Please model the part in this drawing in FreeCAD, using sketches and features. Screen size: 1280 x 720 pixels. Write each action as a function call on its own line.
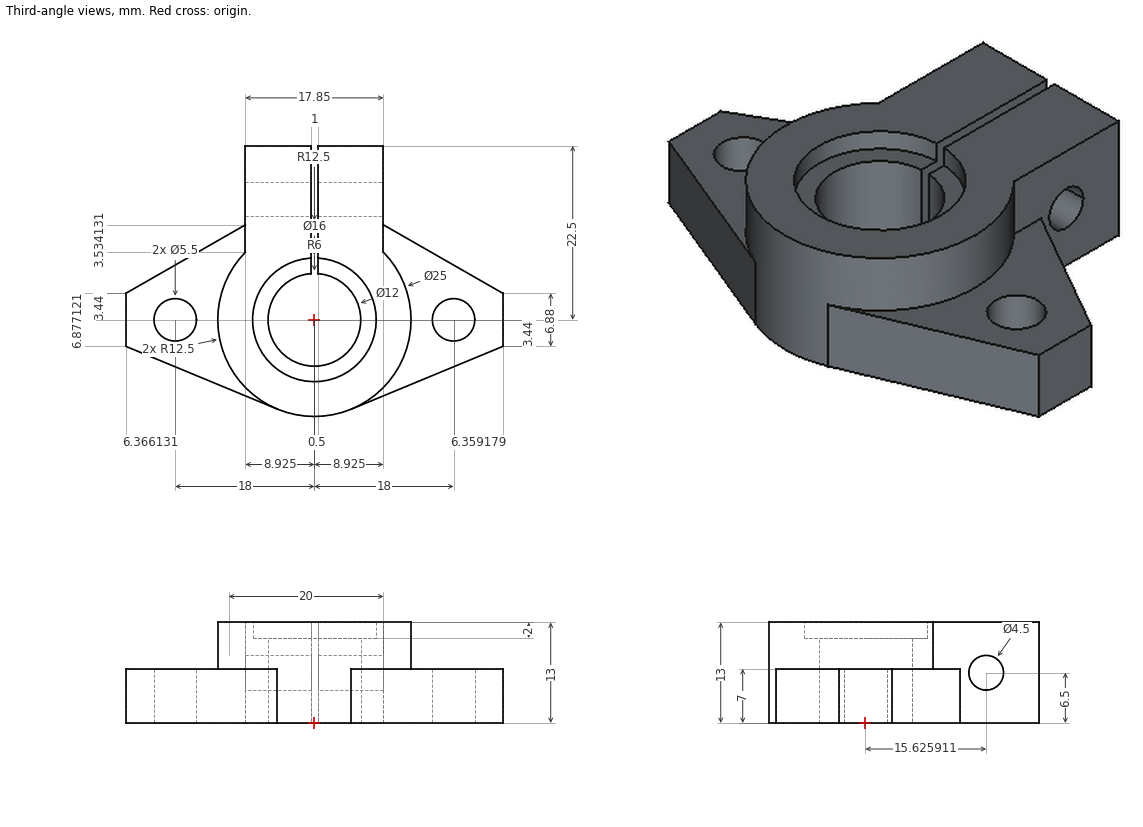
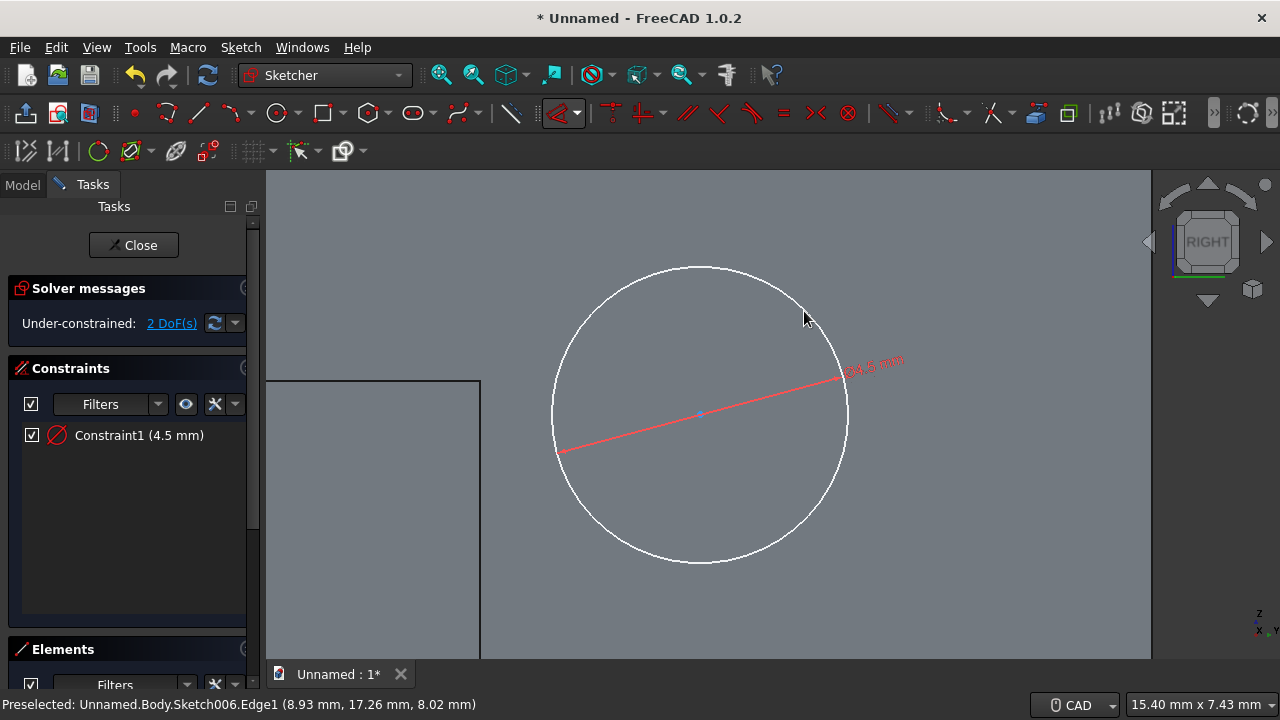
click(700, 415)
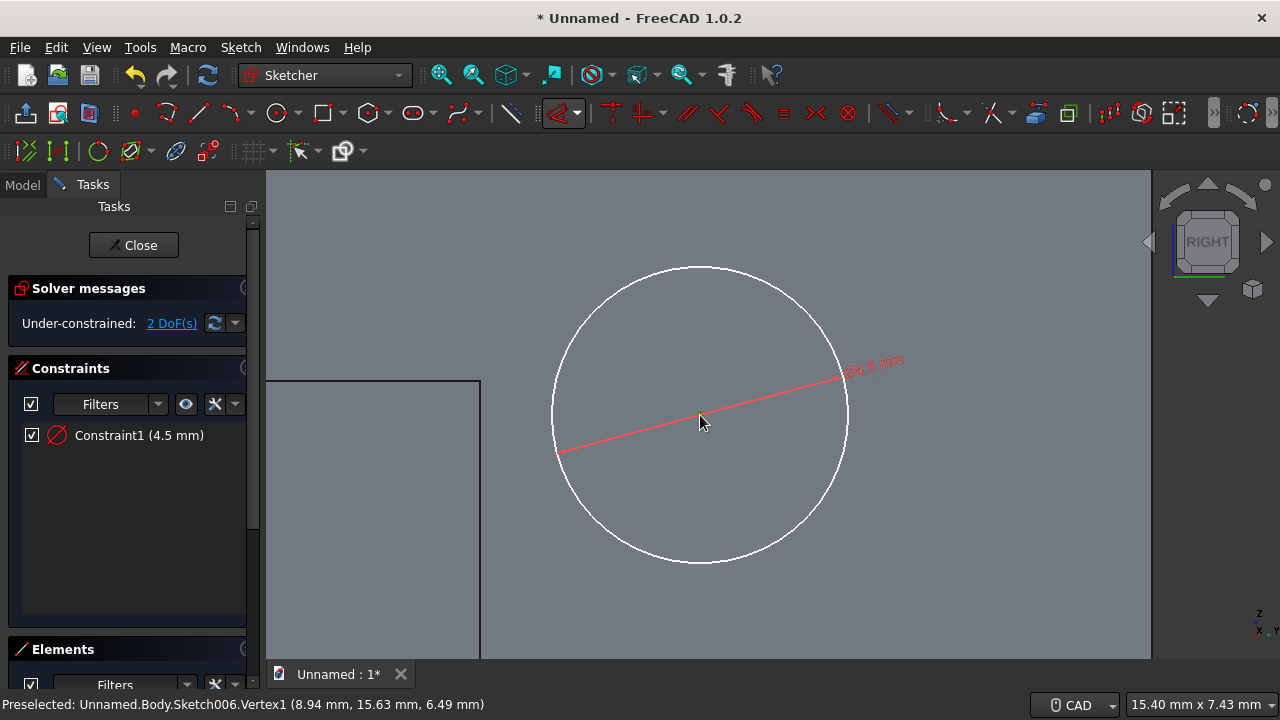
click(580, 114)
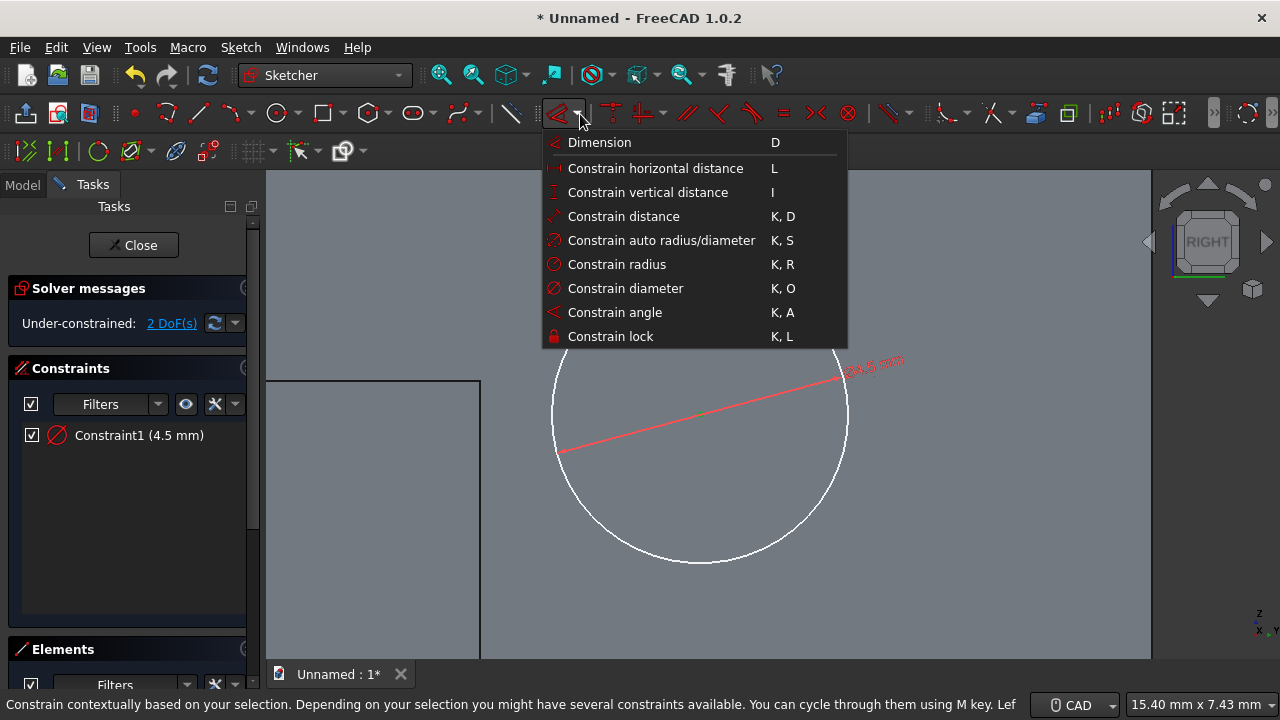
click(695, 192)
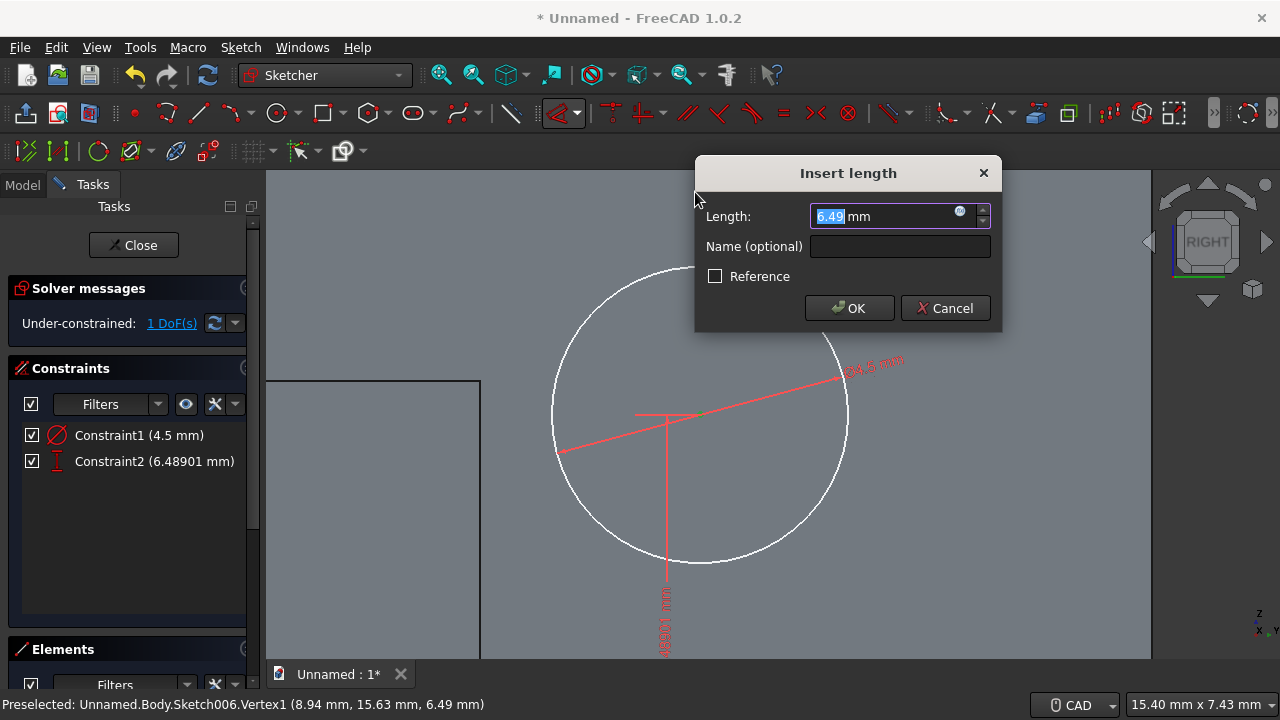
text(6.5)
key(Return)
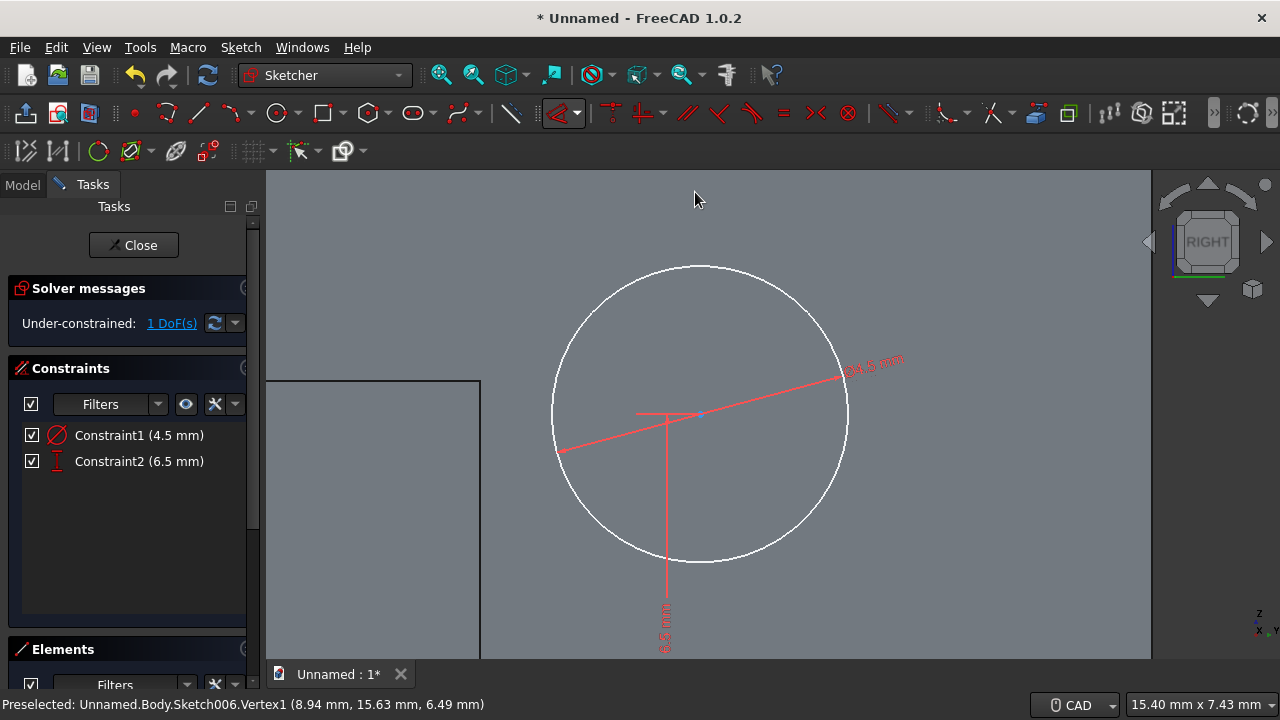
click(700, 414)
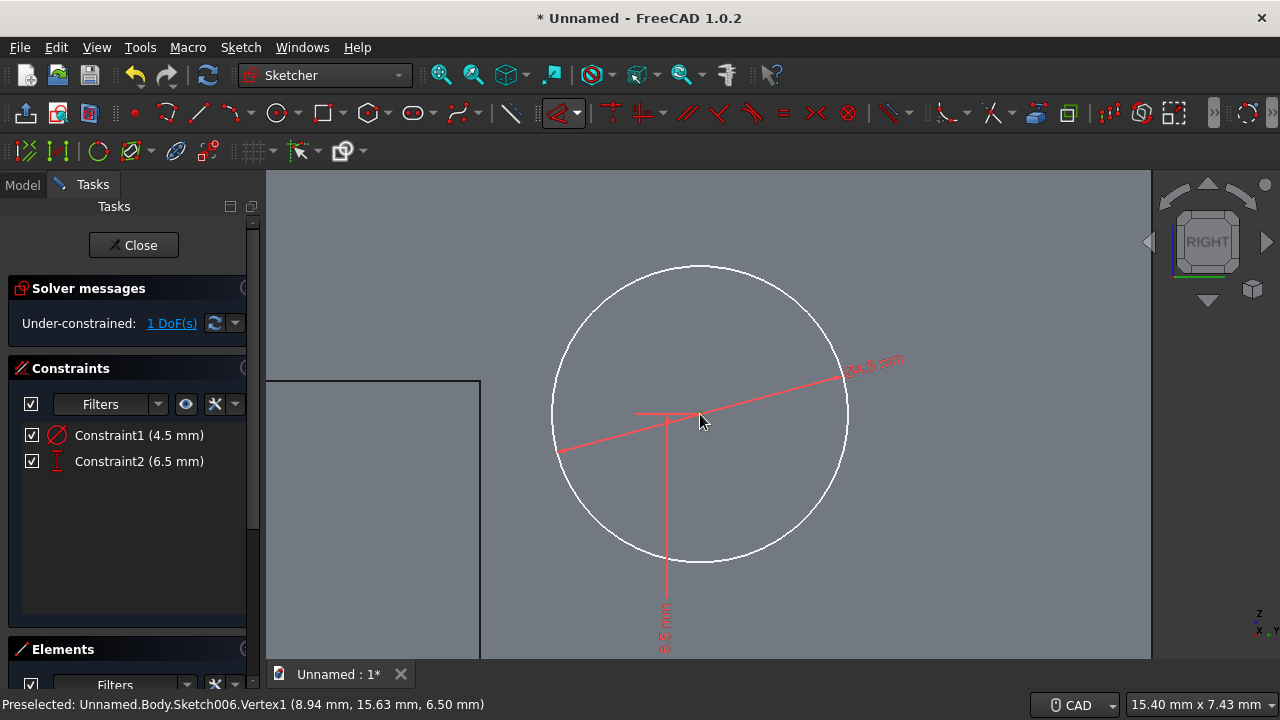
click(580, 114)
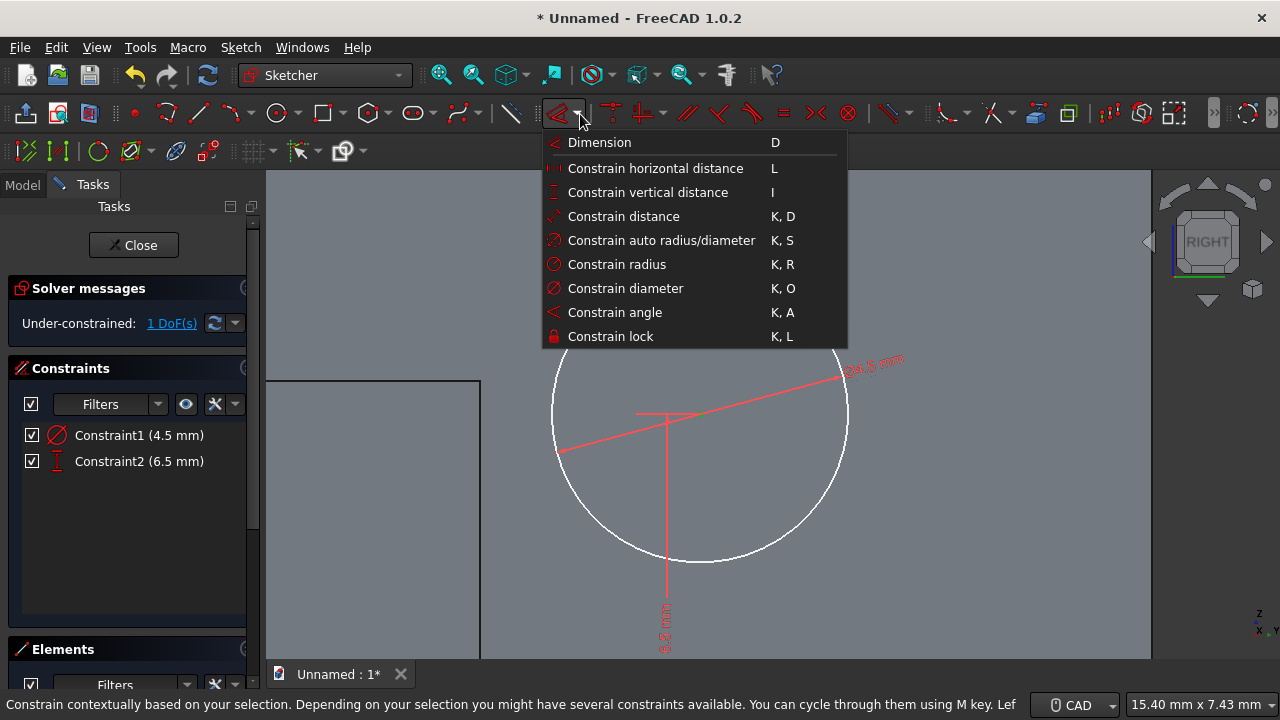
click(695, 168)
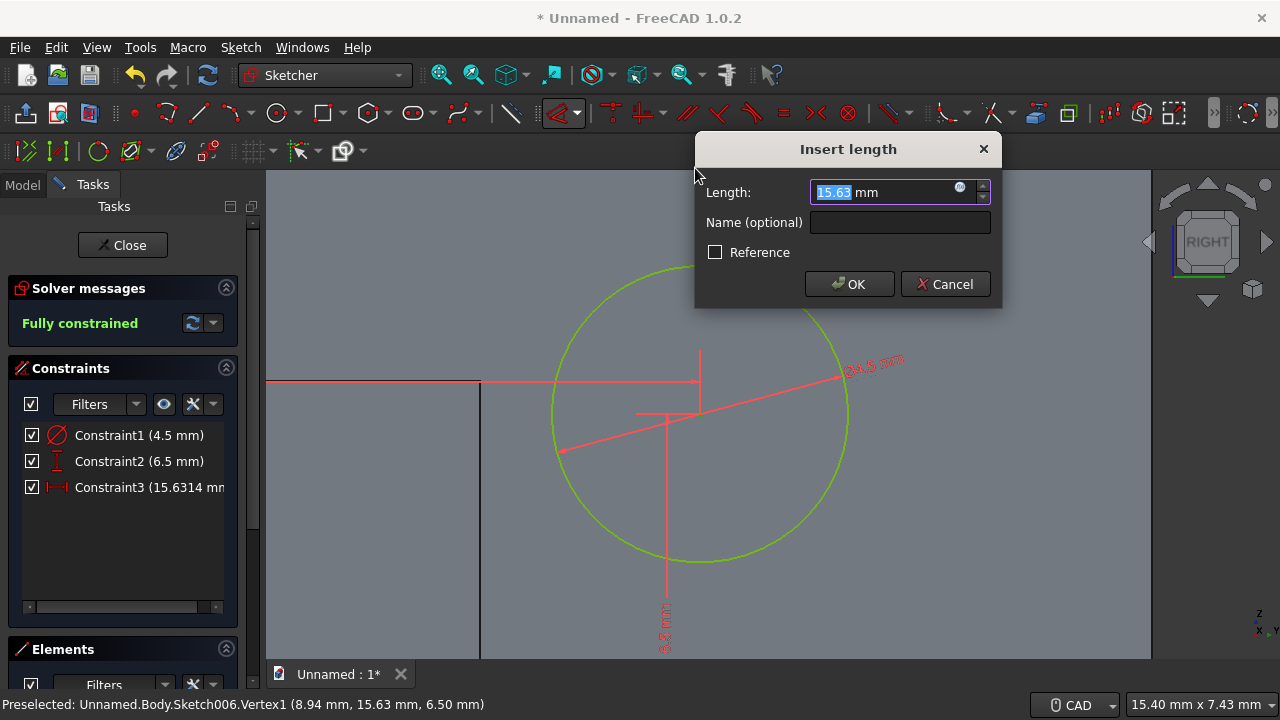
text(15.625911)
key(Return)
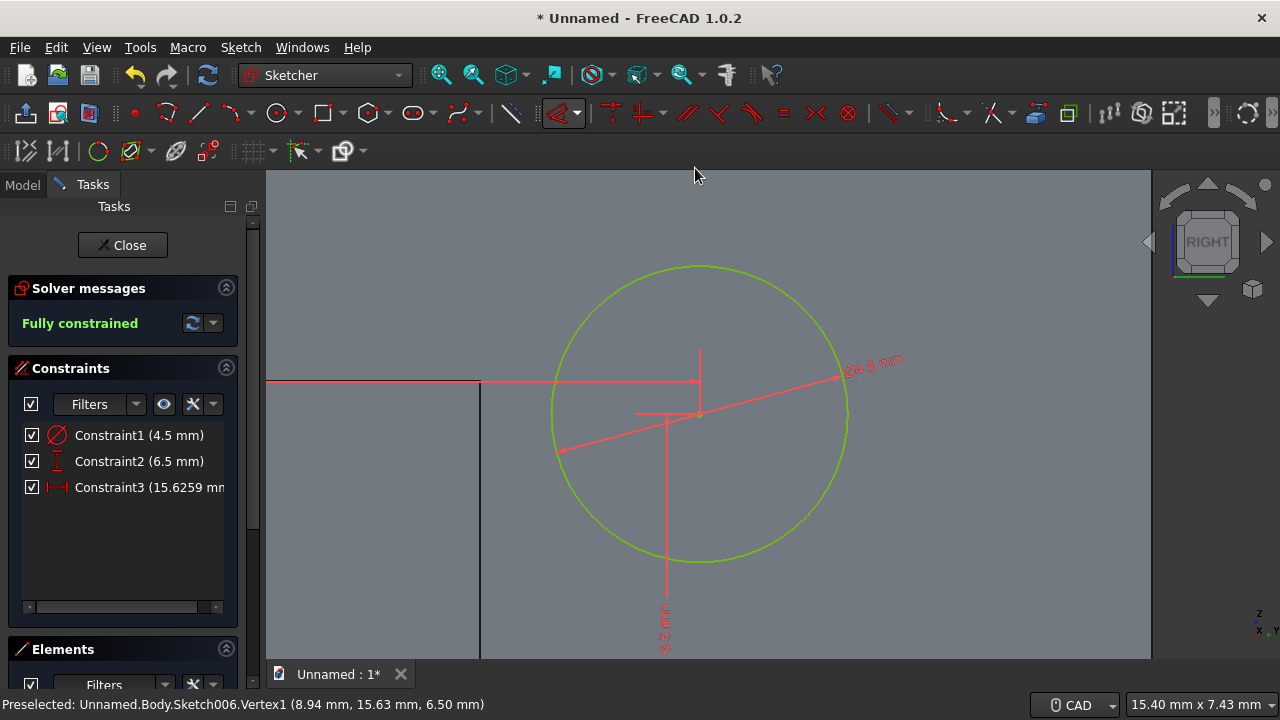
click(123, 245)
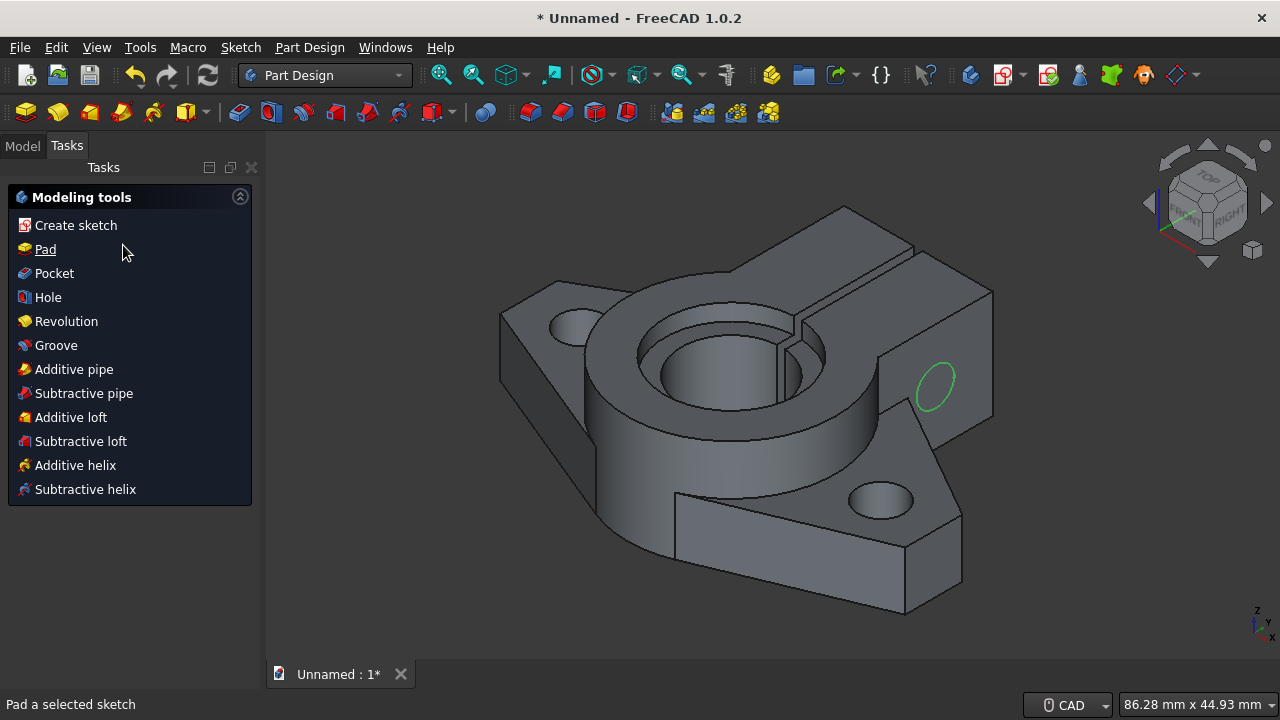
click(240, 112)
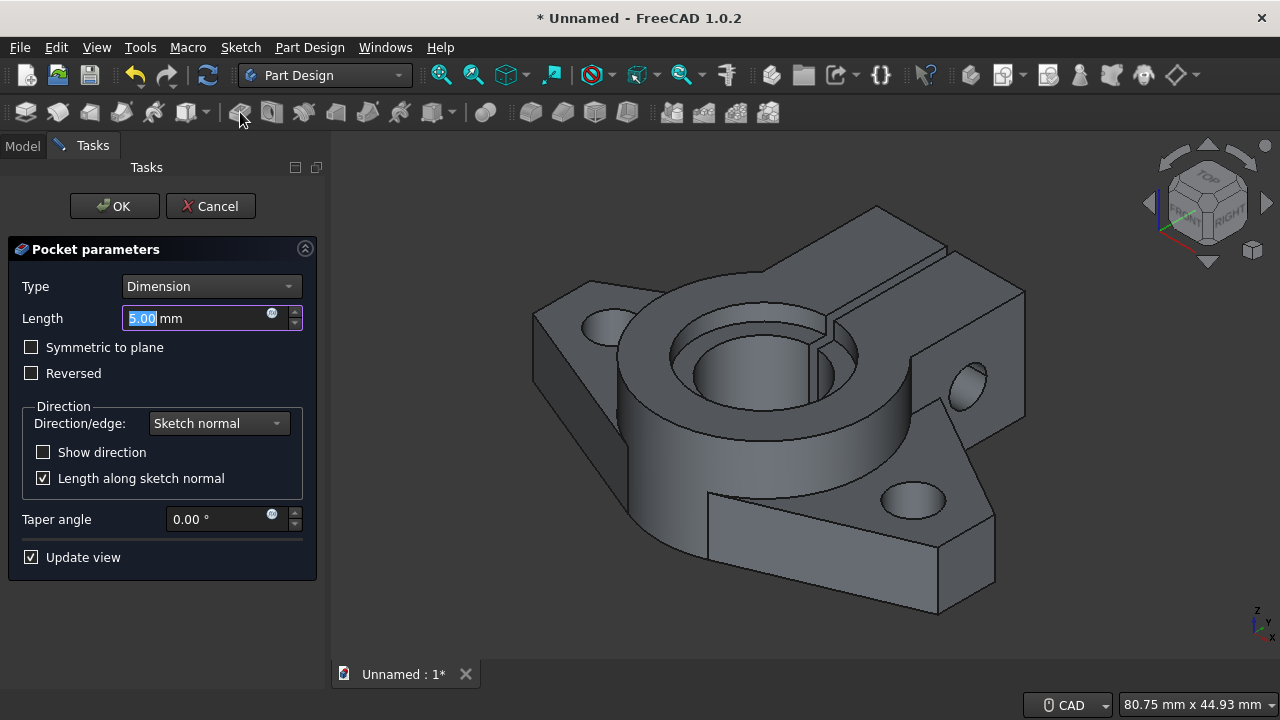
text(20)
key(Tab)